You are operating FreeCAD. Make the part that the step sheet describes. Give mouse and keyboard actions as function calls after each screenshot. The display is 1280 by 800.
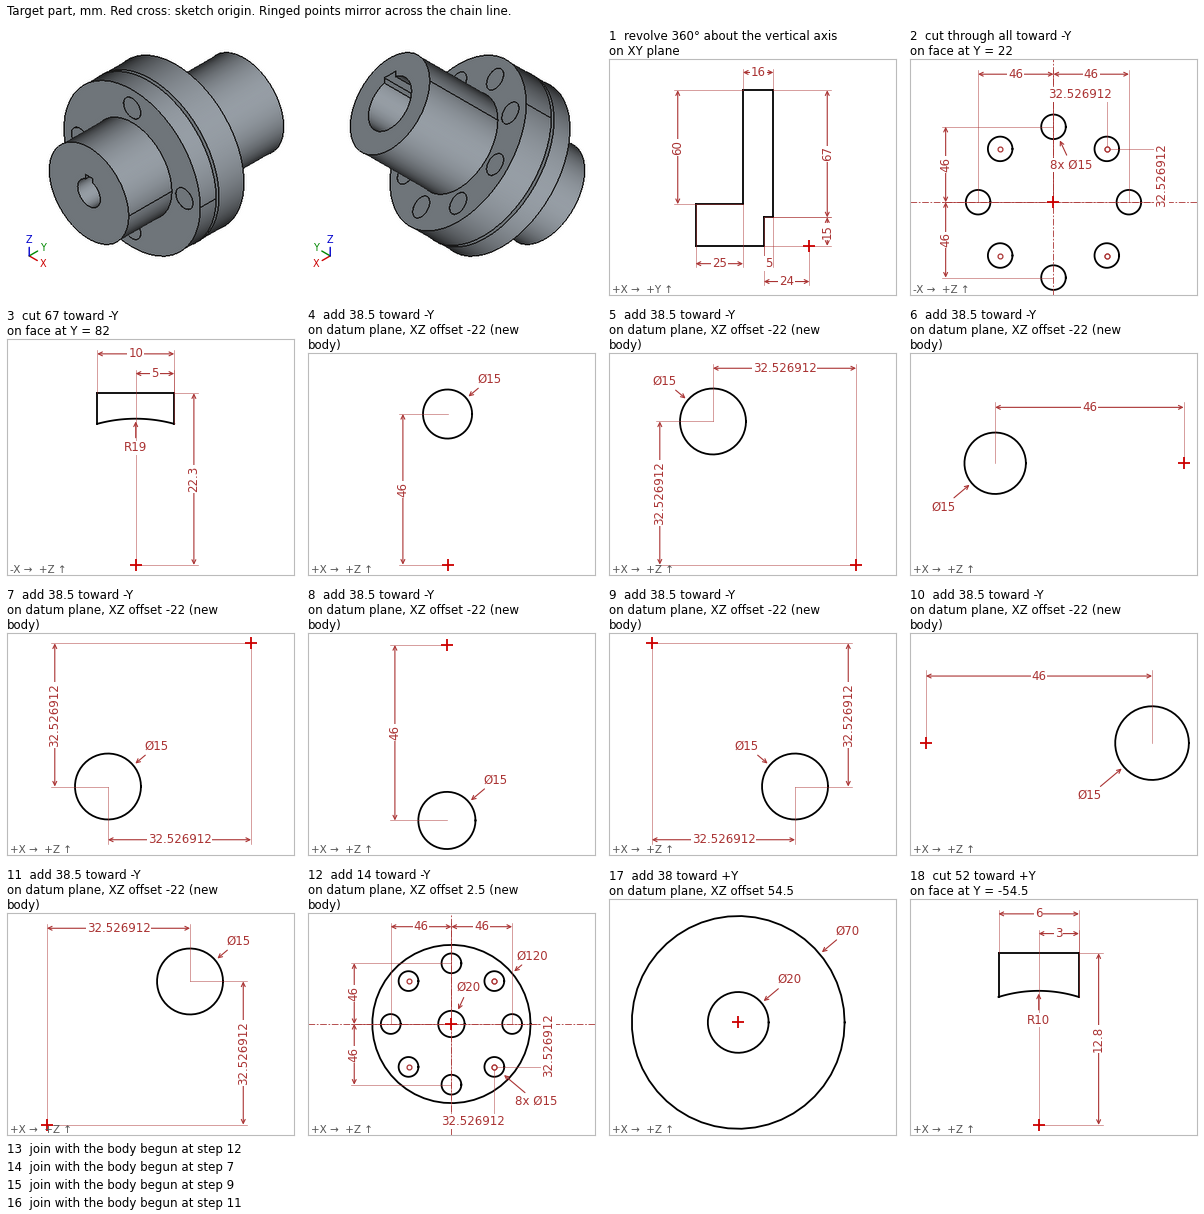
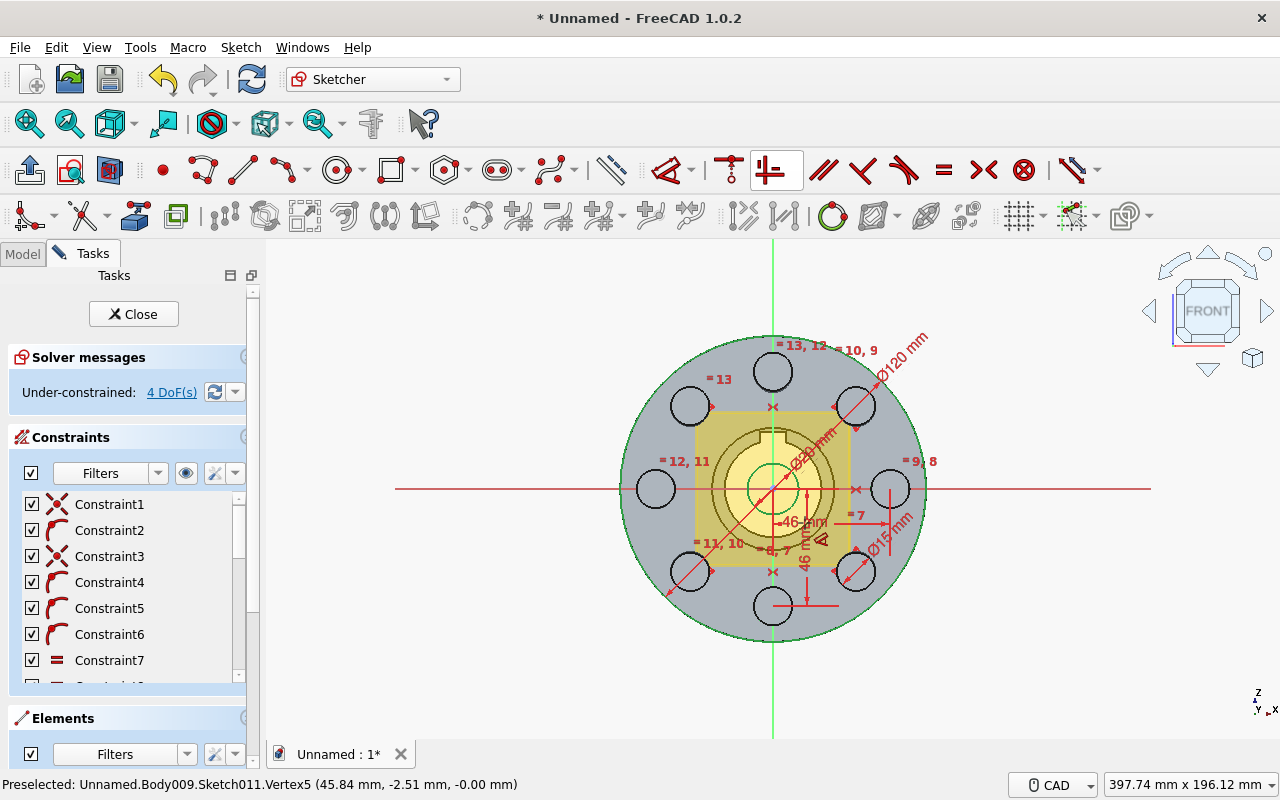
click(656, 489)
click(715, 523)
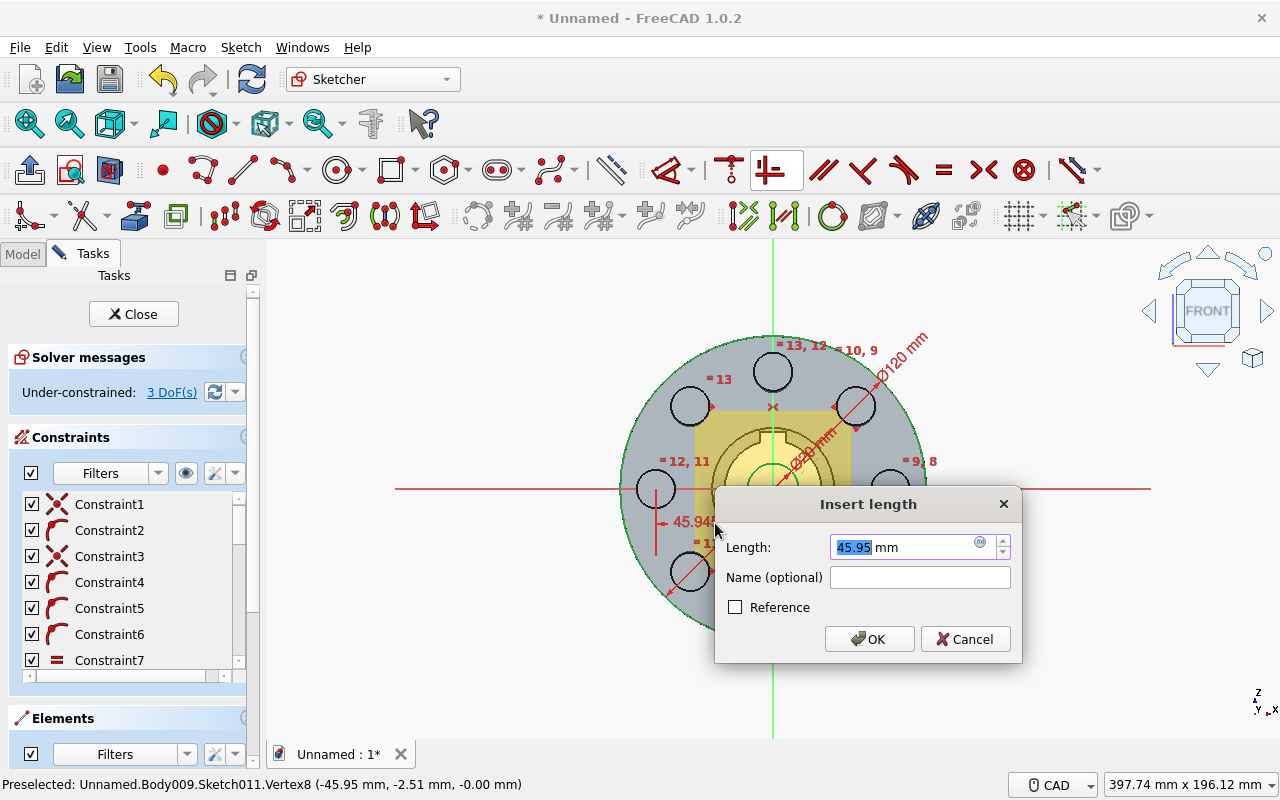
text(46)
key(Return)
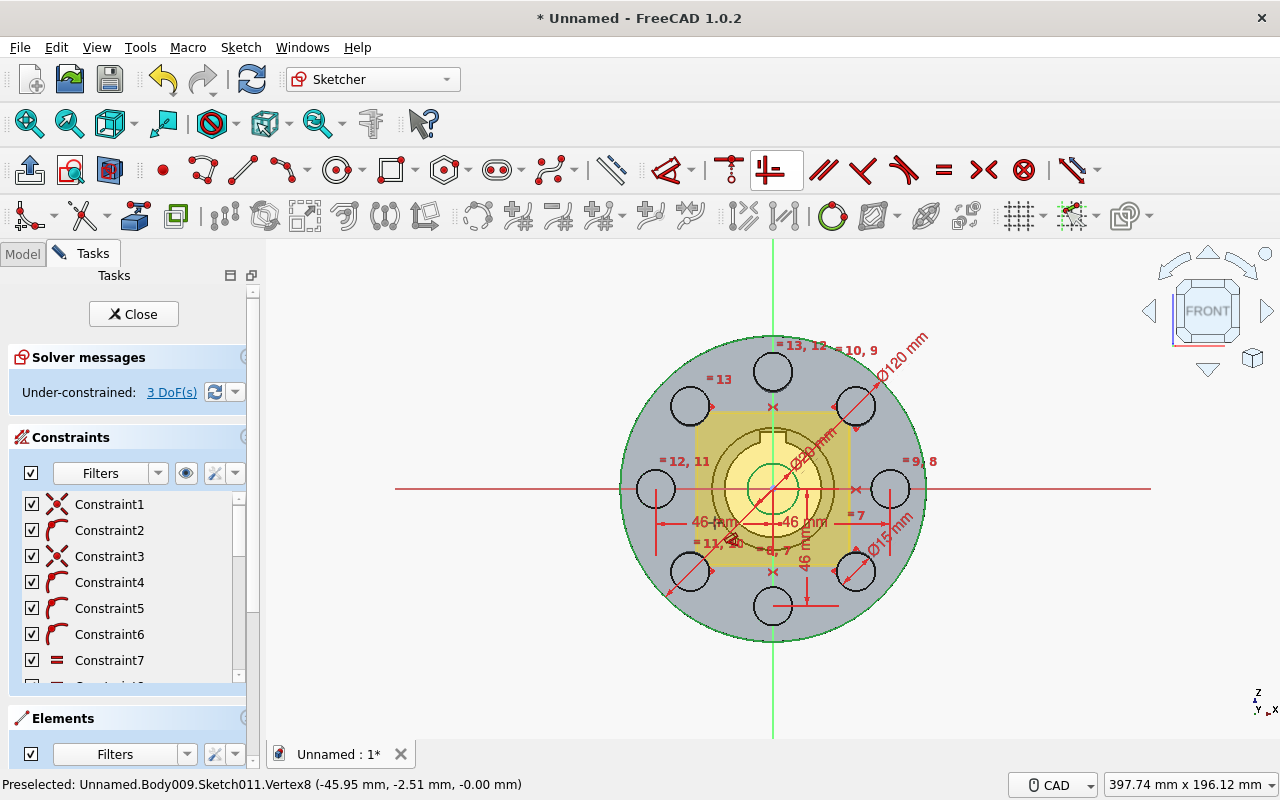
click(773, 373)
click(807, 404)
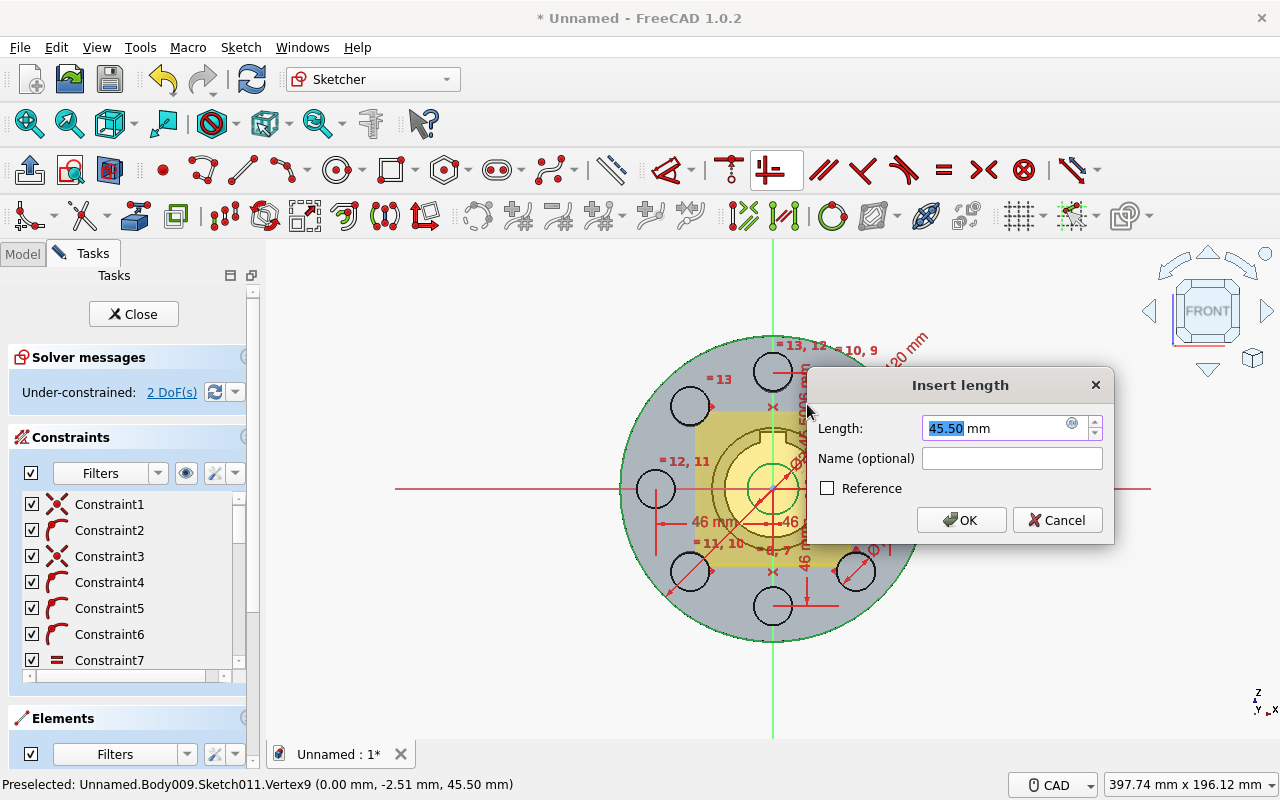
text(46)
key(Return)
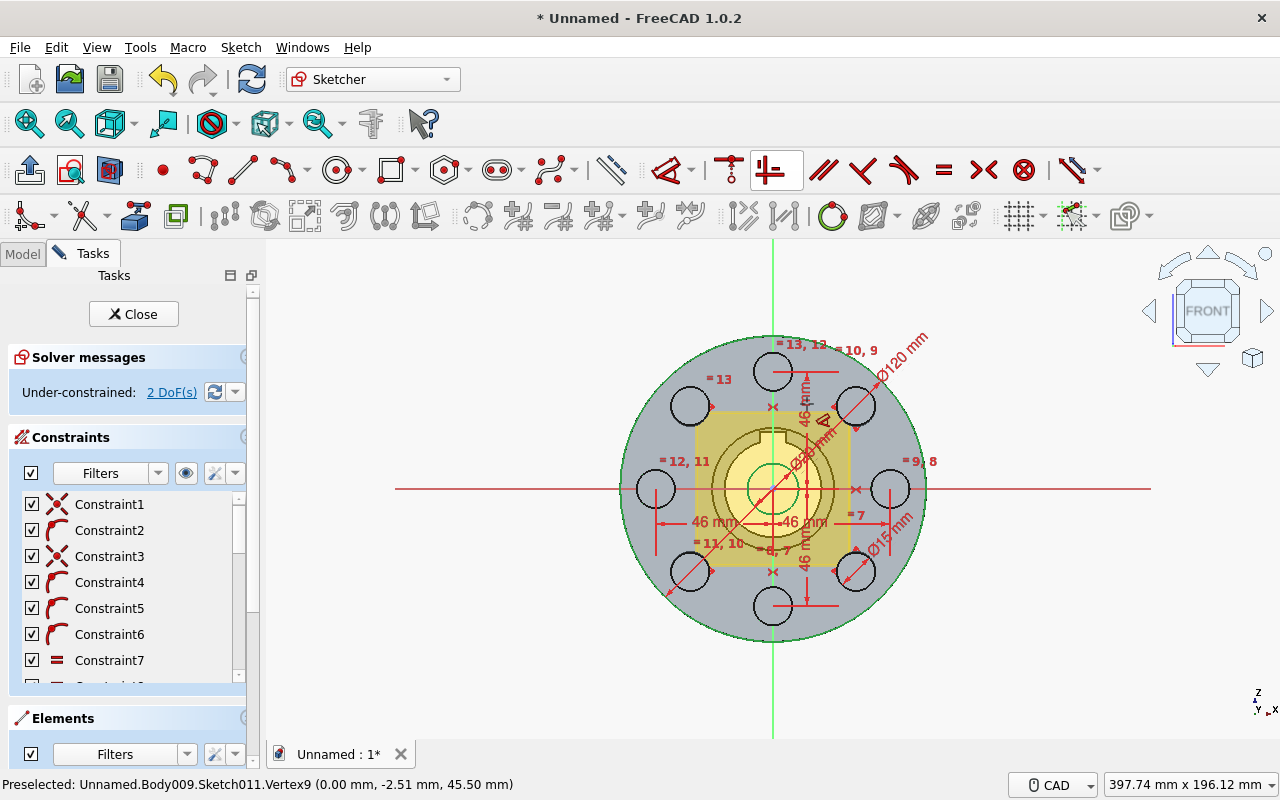
click(856, 571)
click(815, 605)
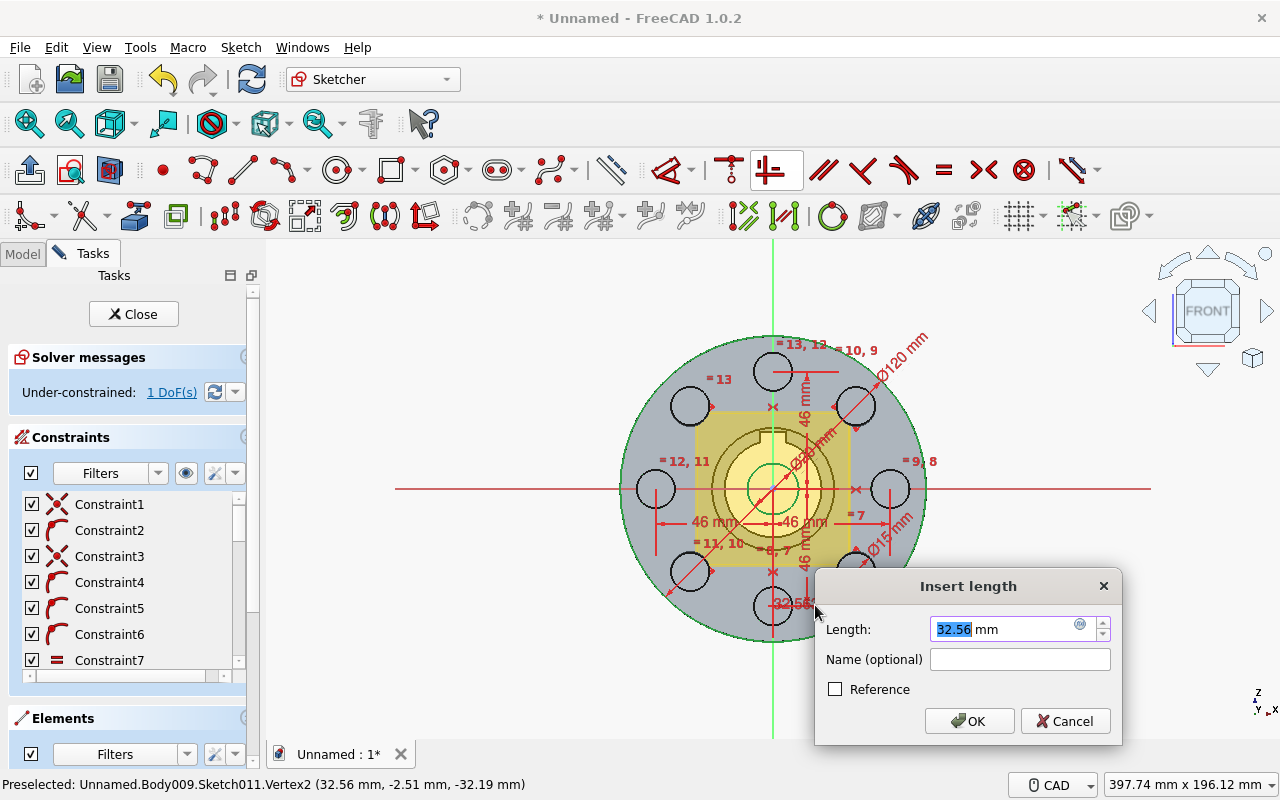
text(32.526912)
key(Return)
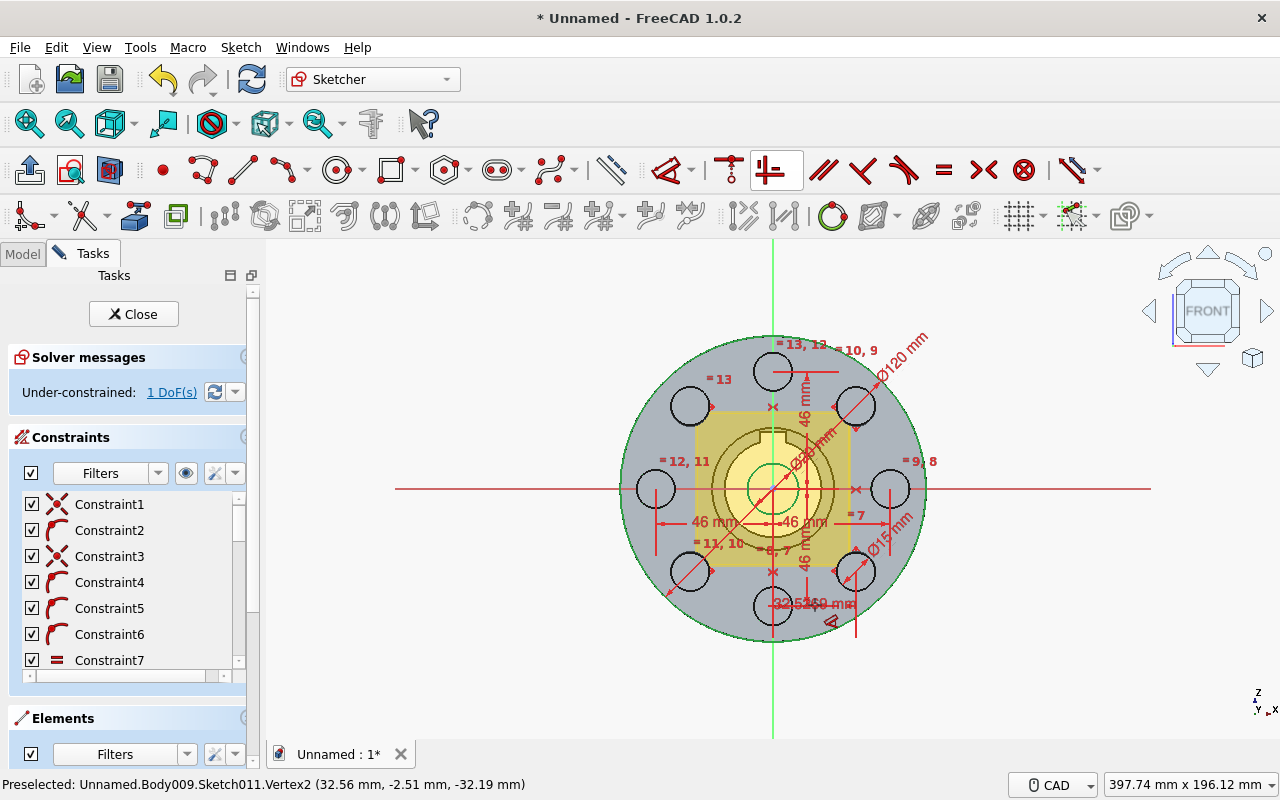
click(856, 571)
click(890, 559)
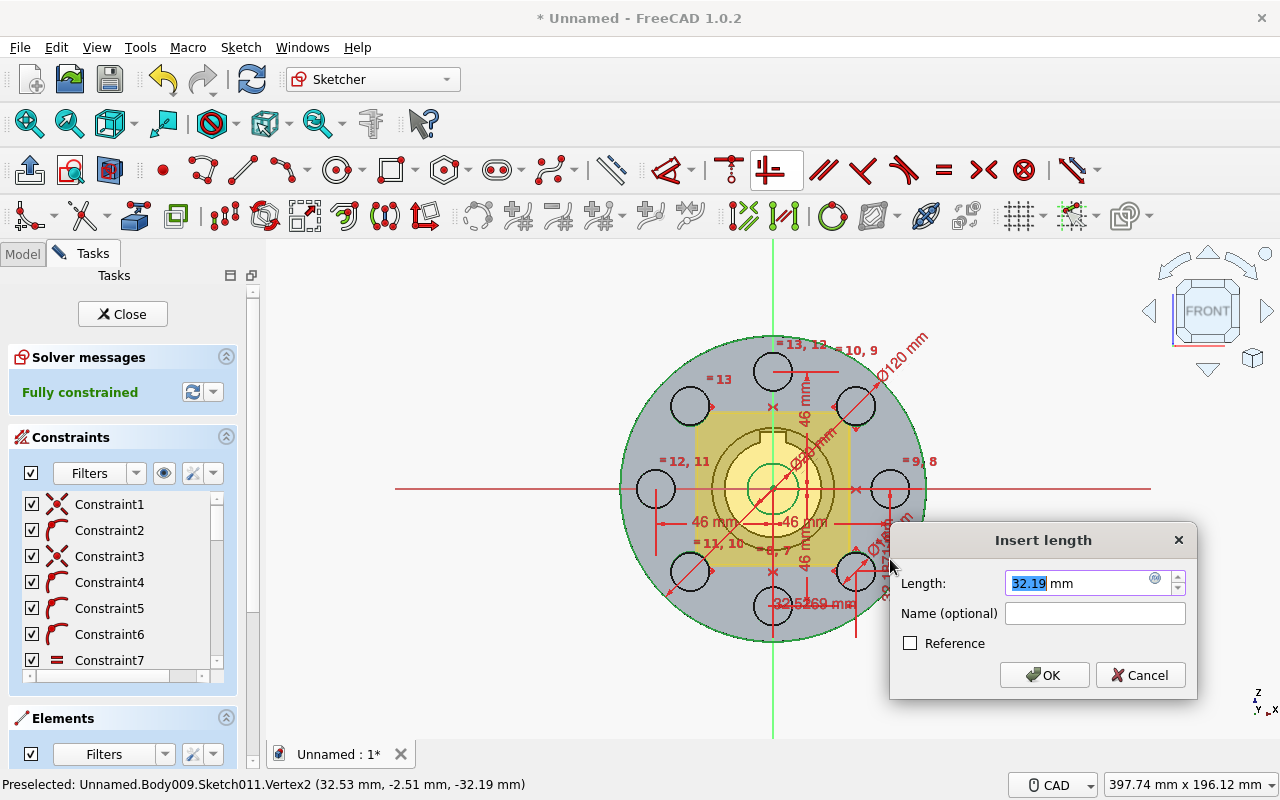
text(32.526912)
key(Return)
key(Escape)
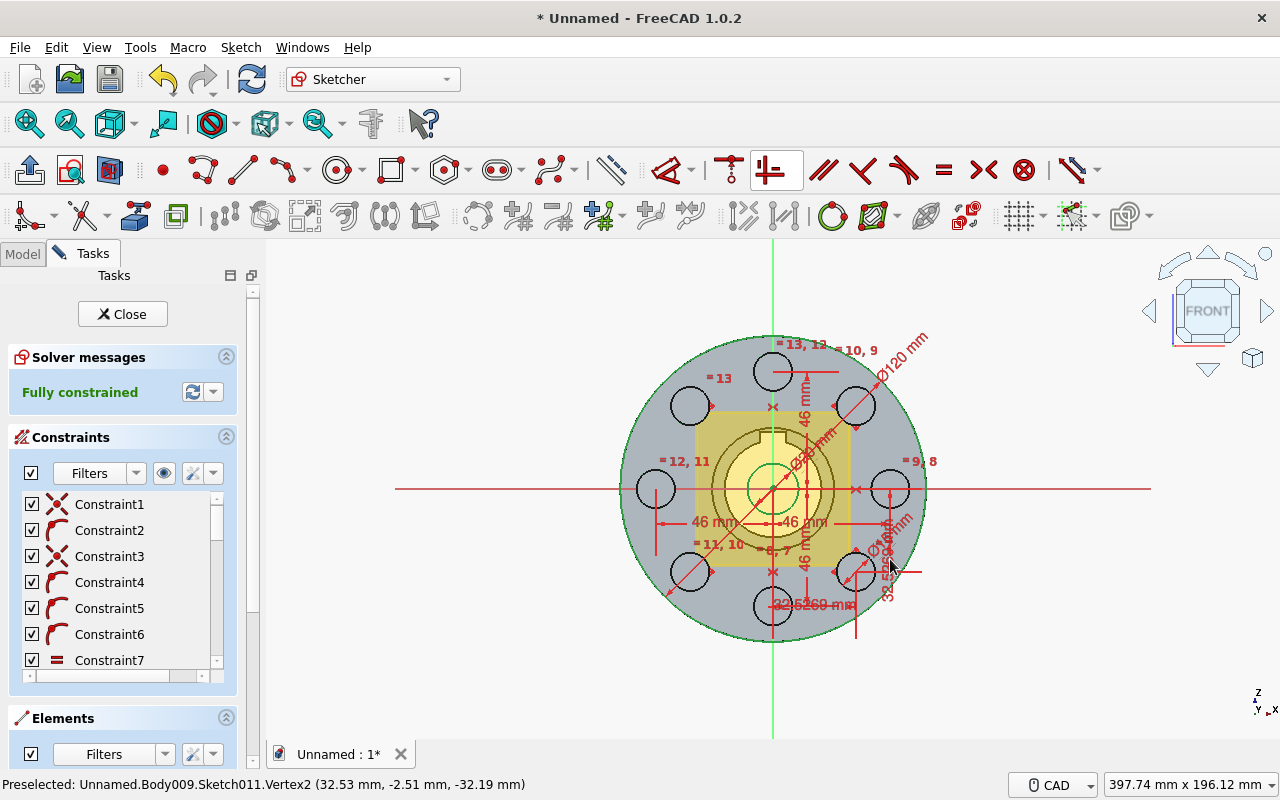
click(123, 314)